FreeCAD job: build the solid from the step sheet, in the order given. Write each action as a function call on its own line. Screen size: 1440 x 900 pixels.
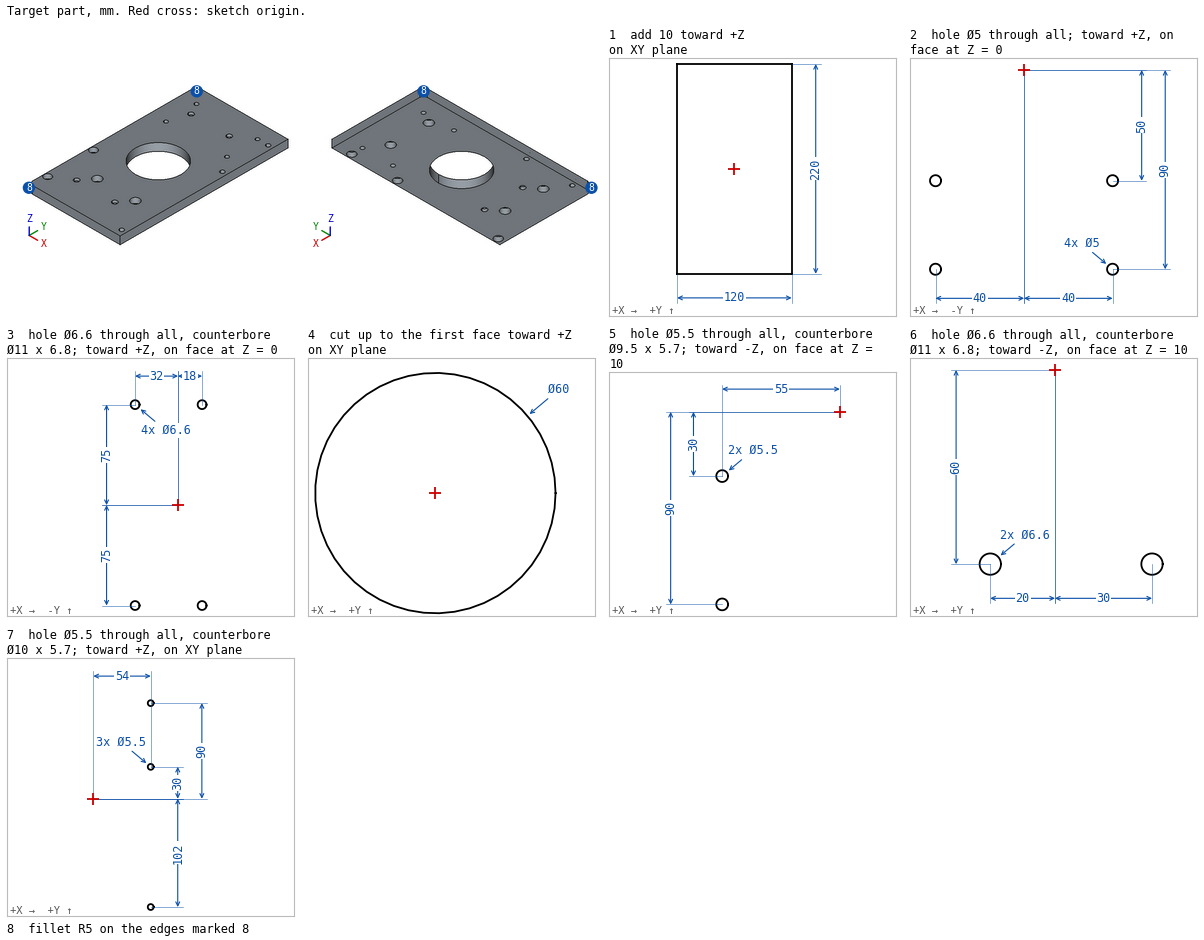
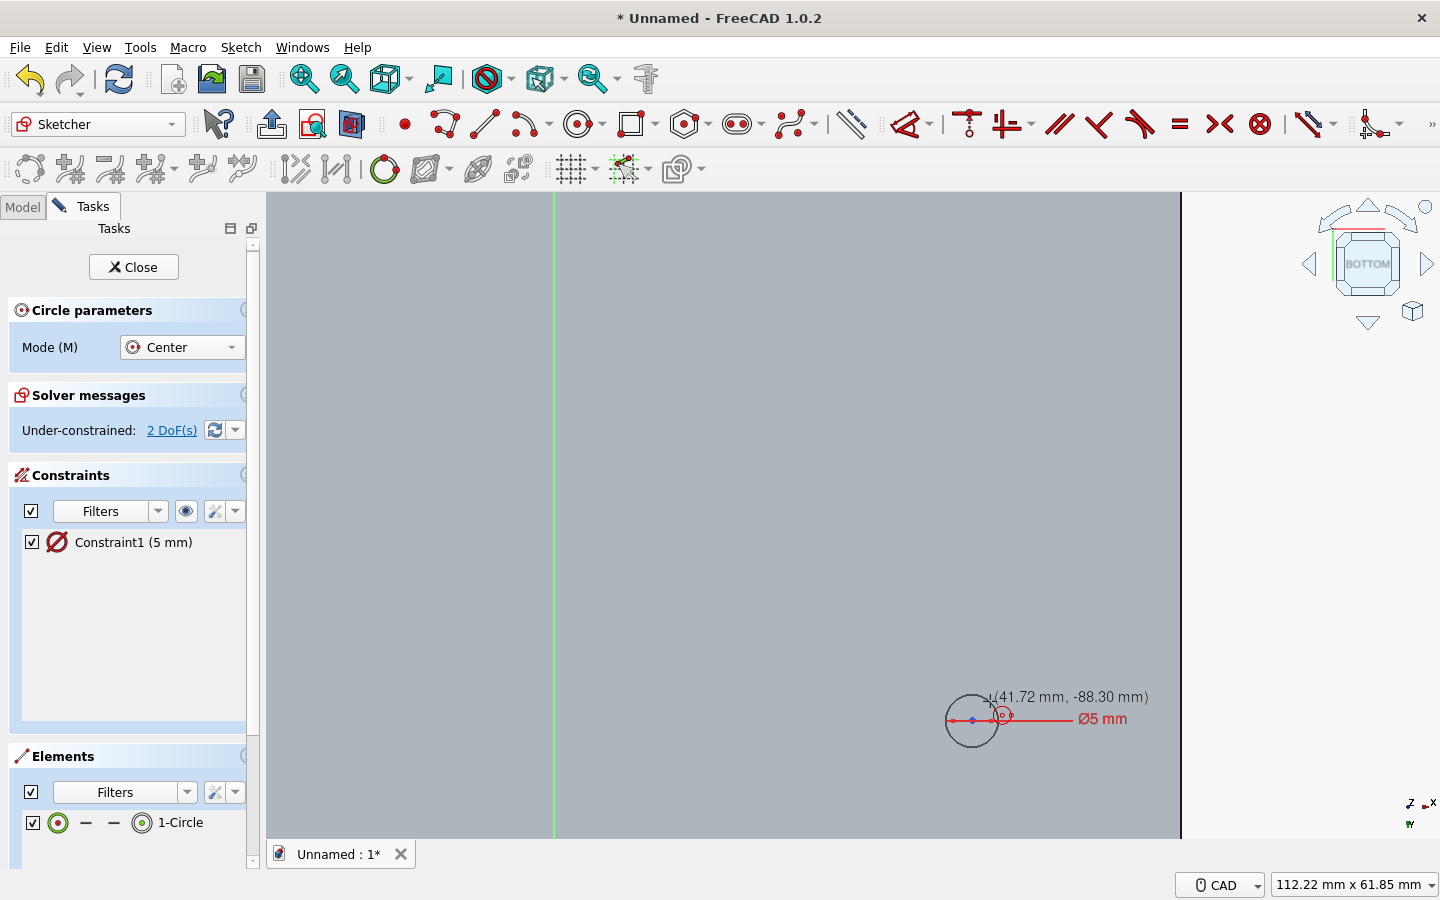
click(972, 301)
move(990, 283)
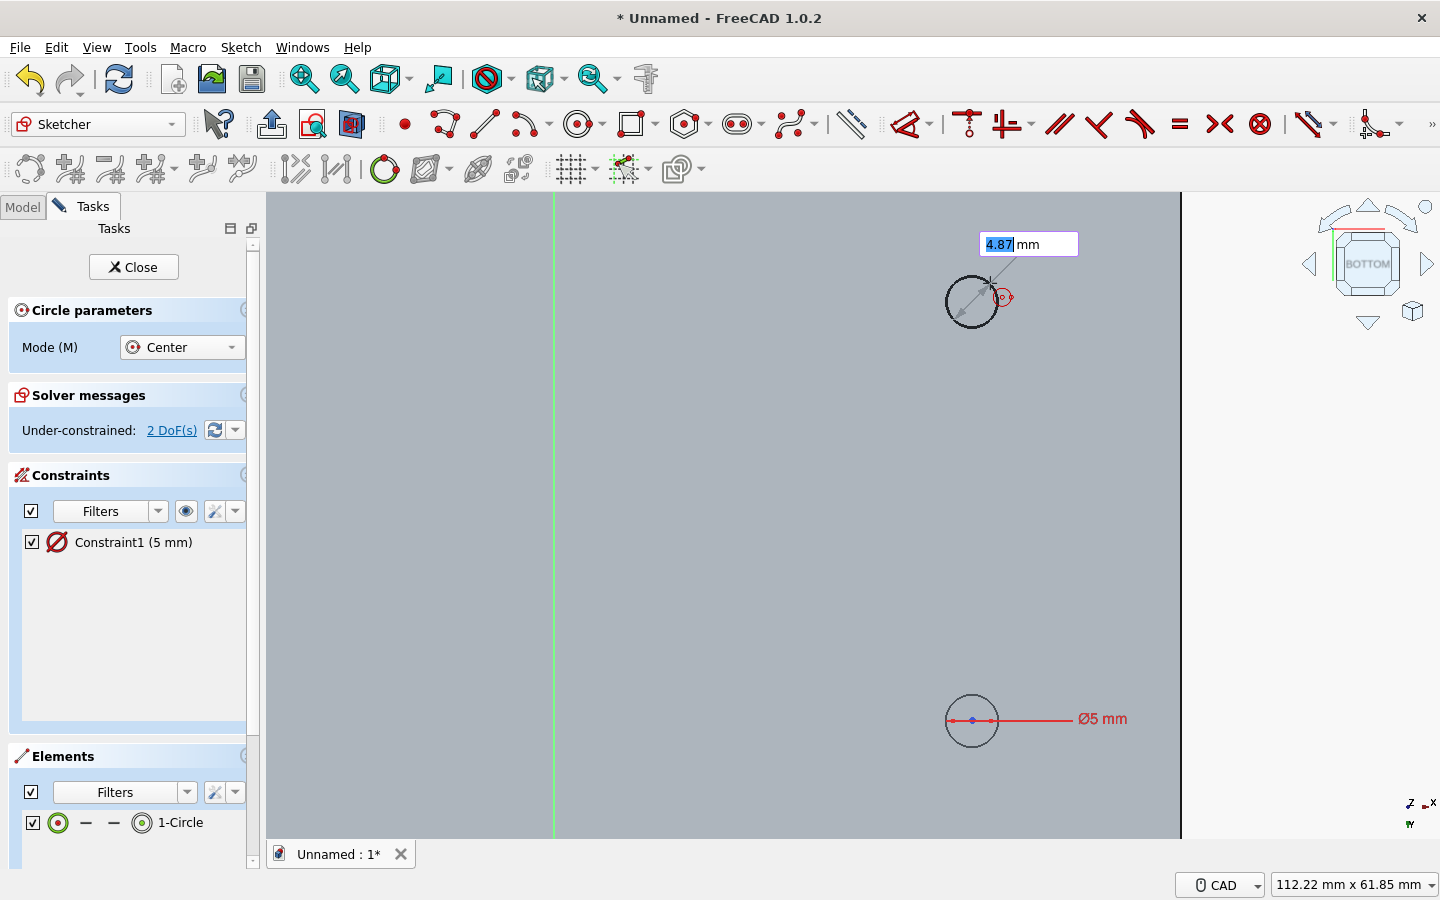
text(5)
key(Return)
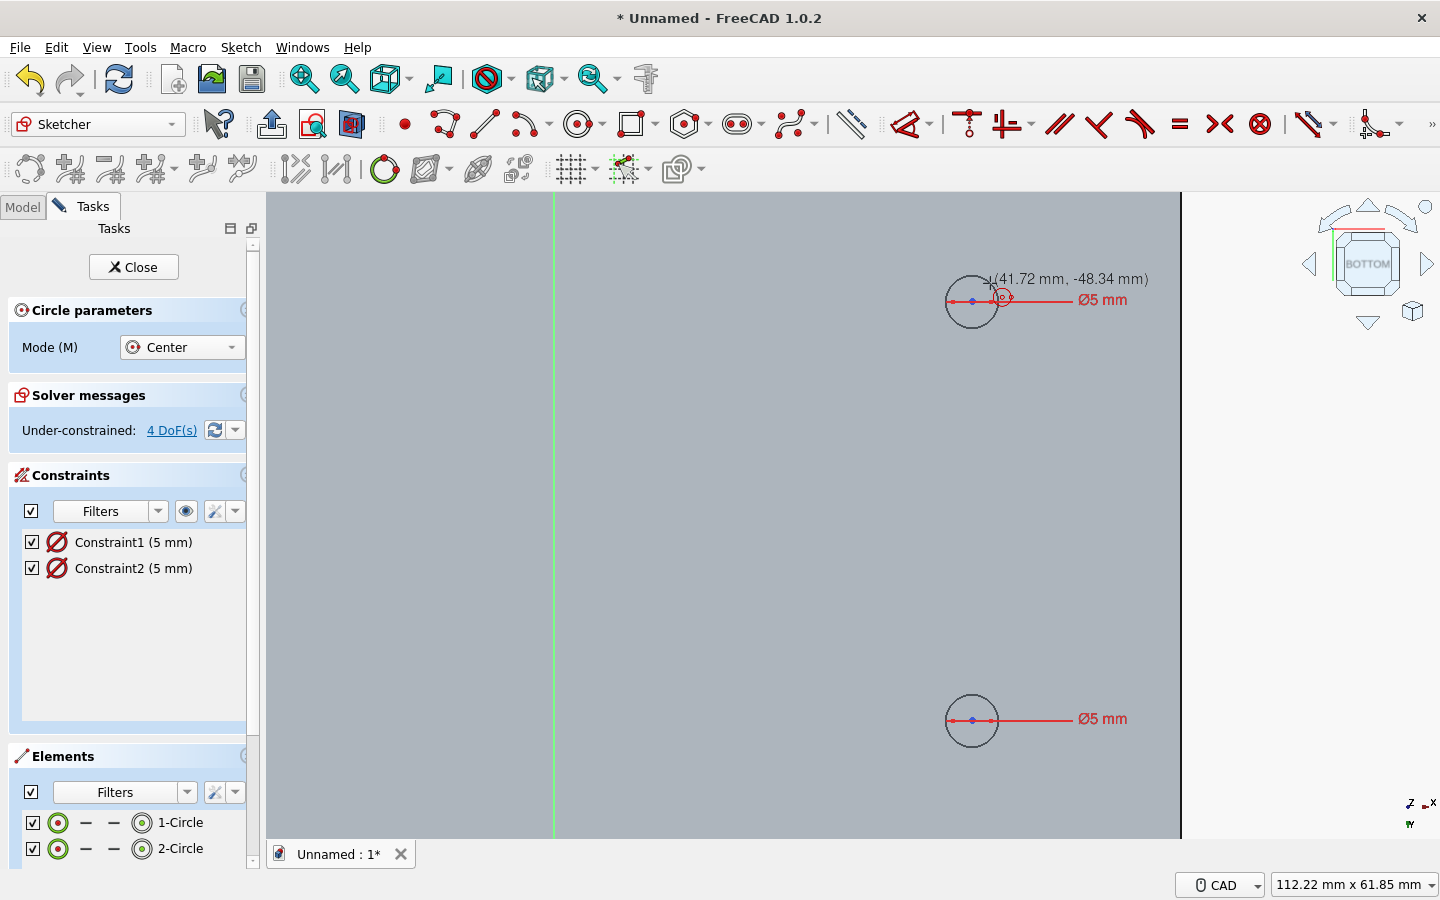
scroll(973, 722, down, 4)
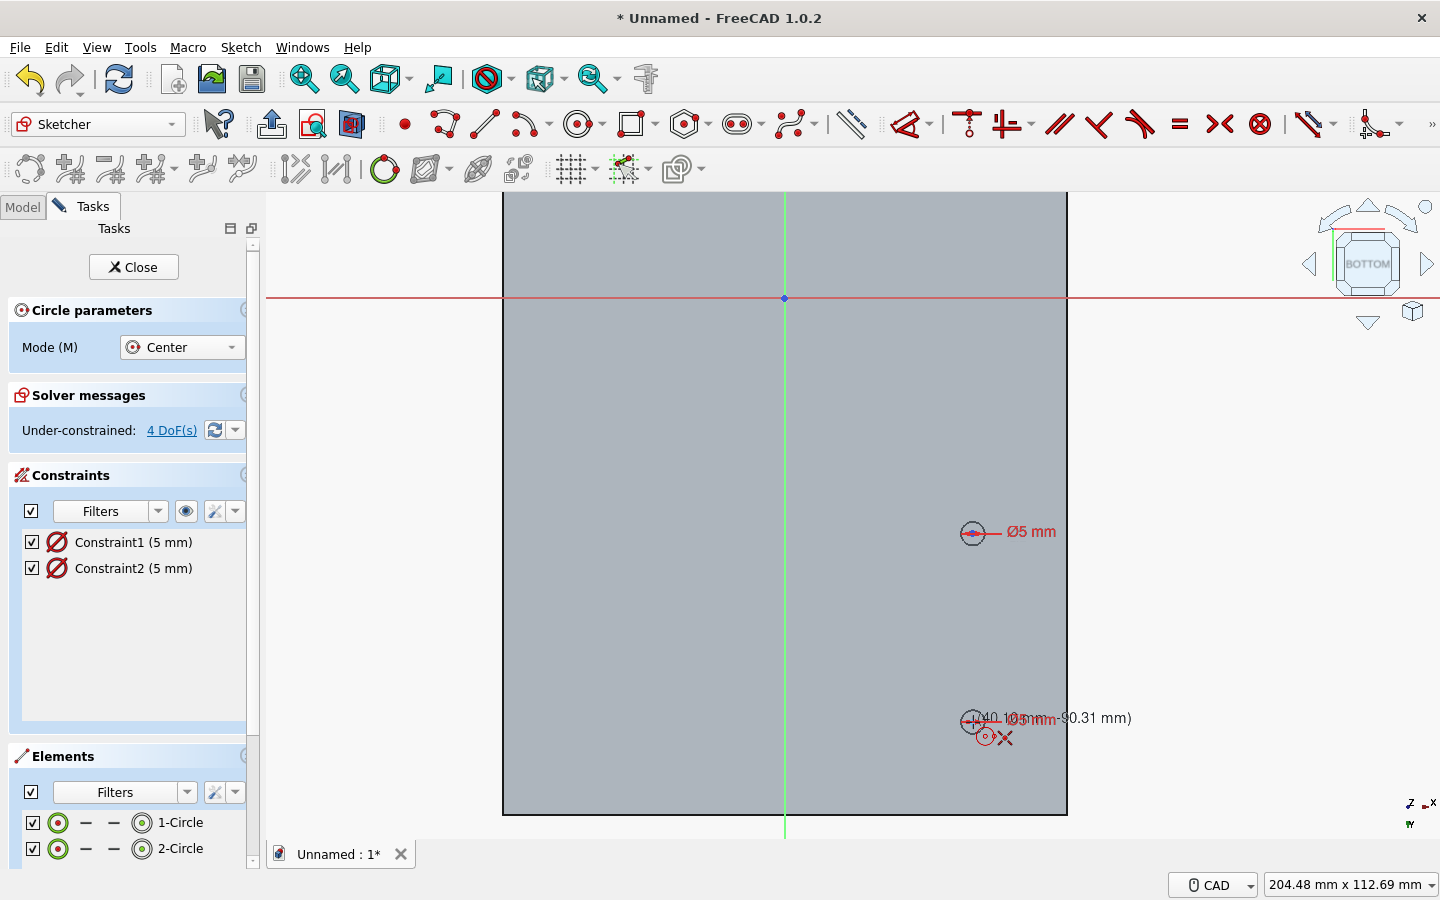
scroll(597, 721, up, 4)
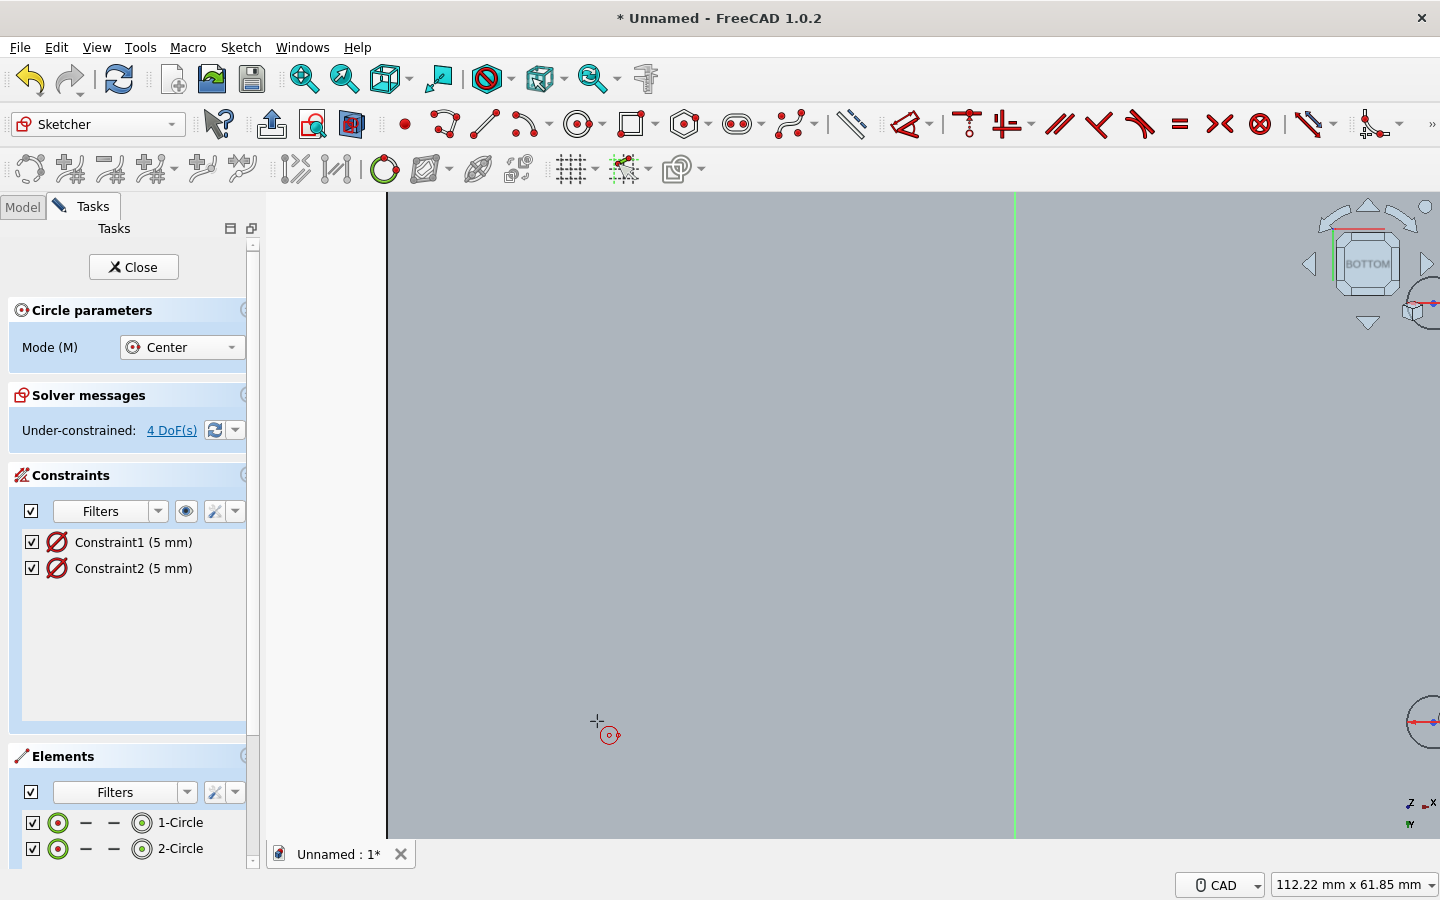
click(596, 721)
move(615, 703)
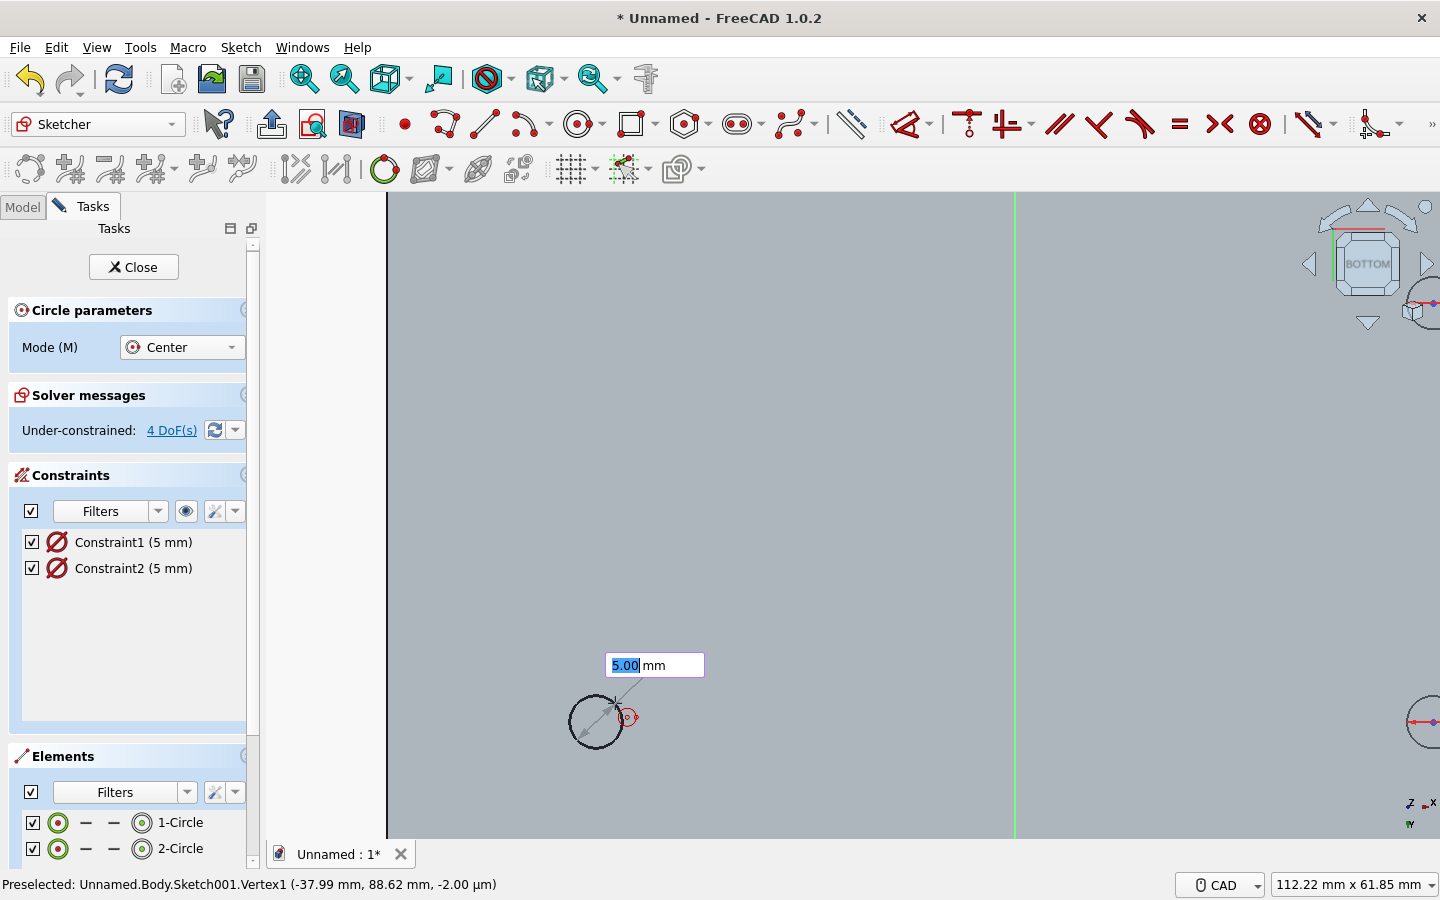
text(5)
key(Return)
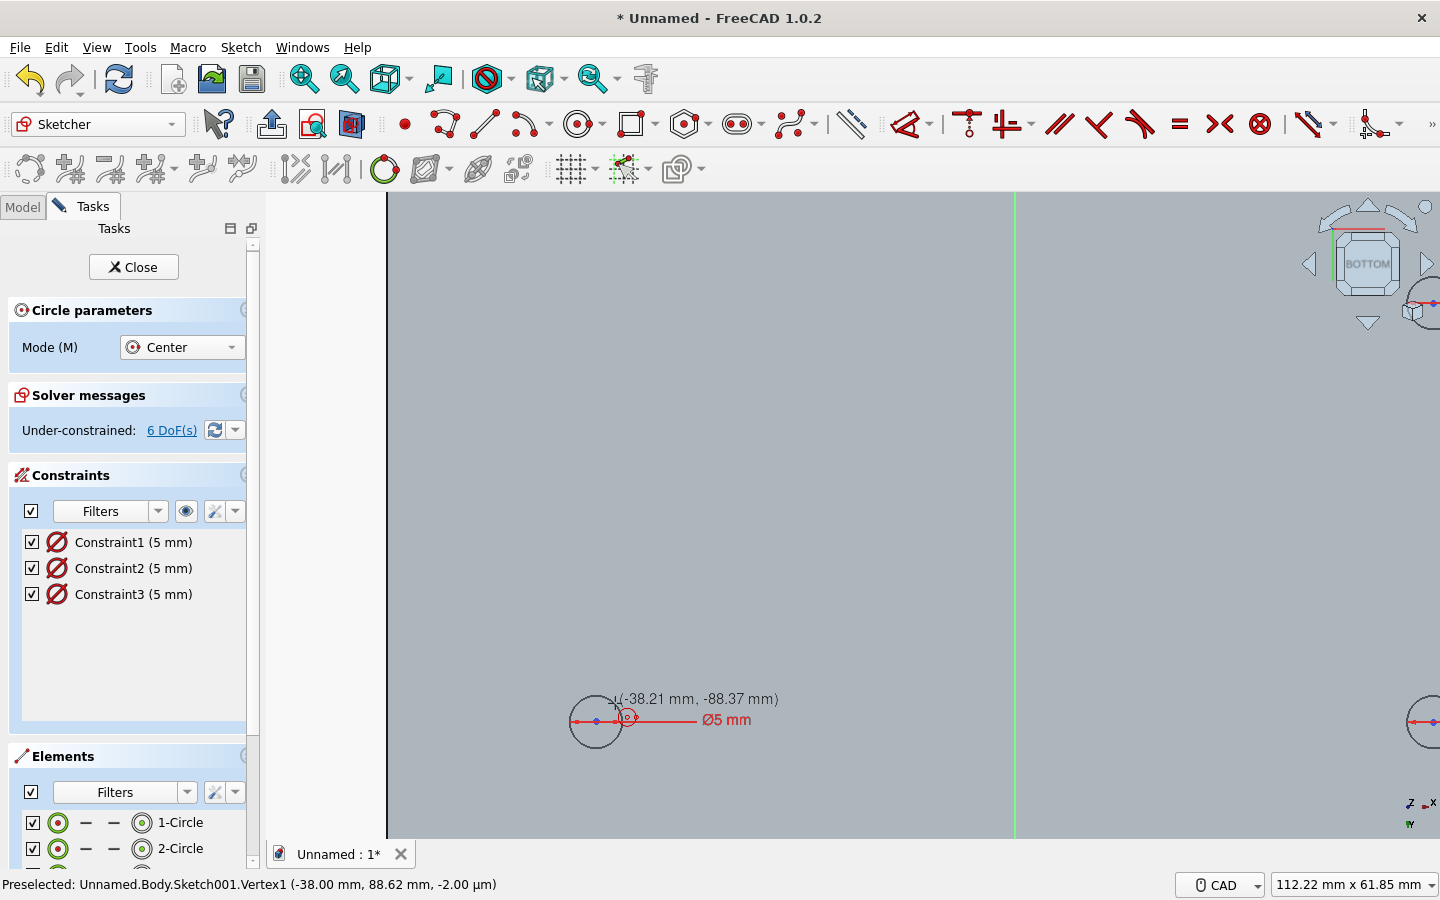
click(596, 303)
move(615, 284)